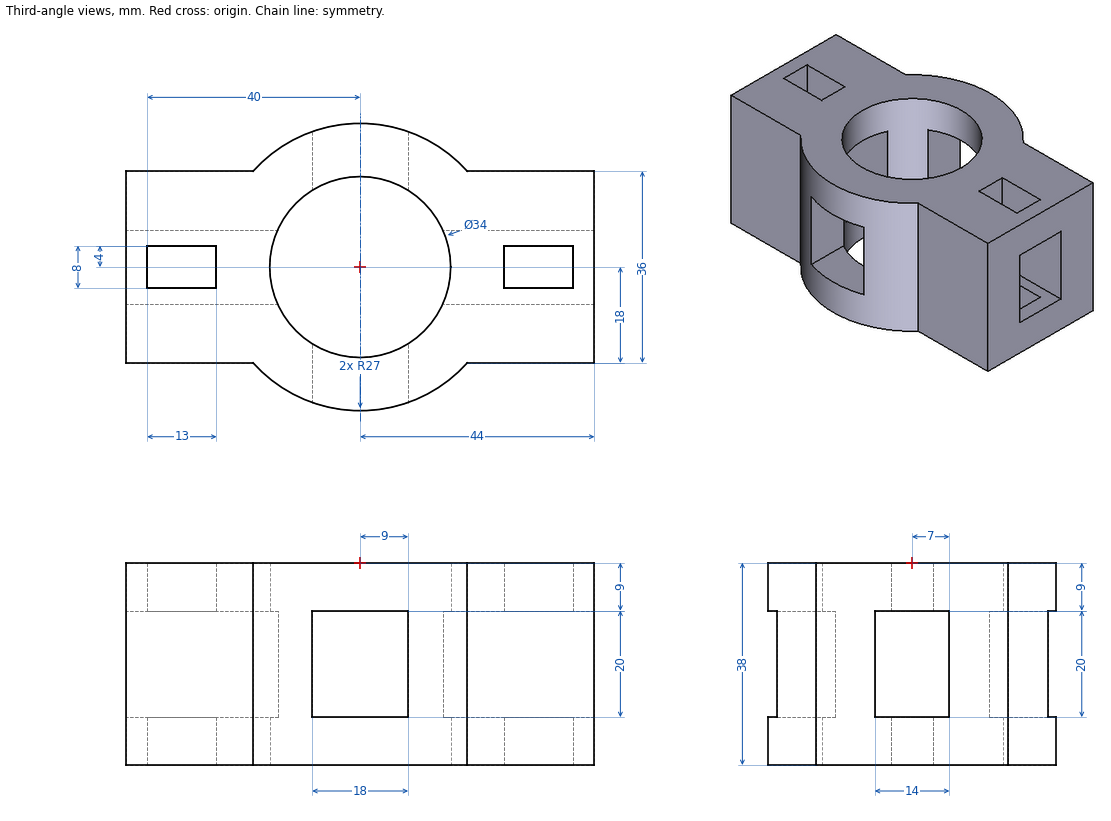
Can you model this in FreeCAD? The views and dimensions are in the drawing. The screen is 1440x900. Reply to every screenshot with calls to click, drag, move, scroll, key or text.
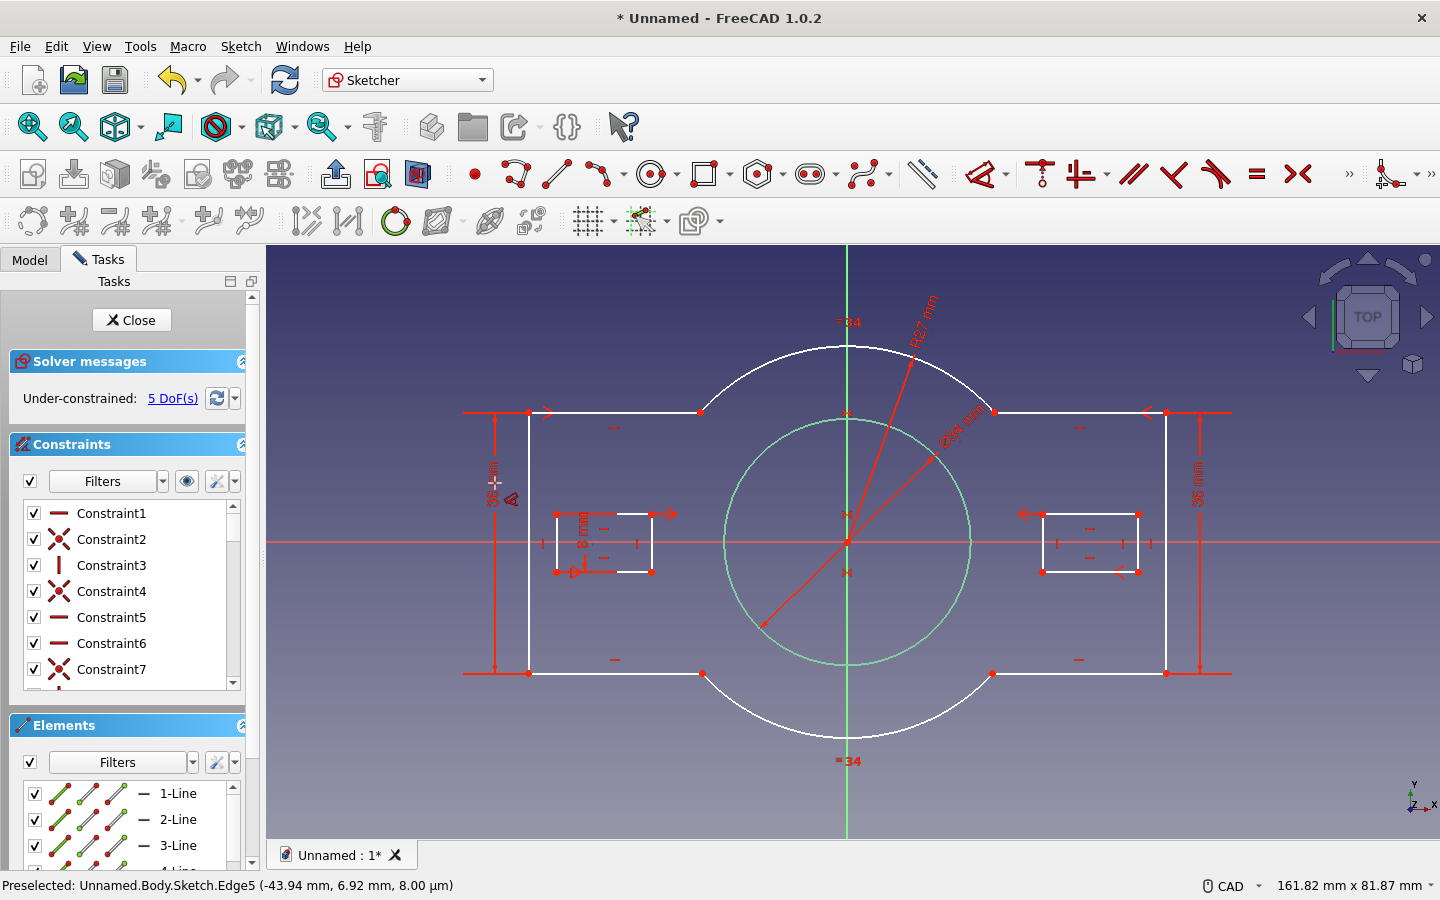
click(585, 572)
click(604, 606)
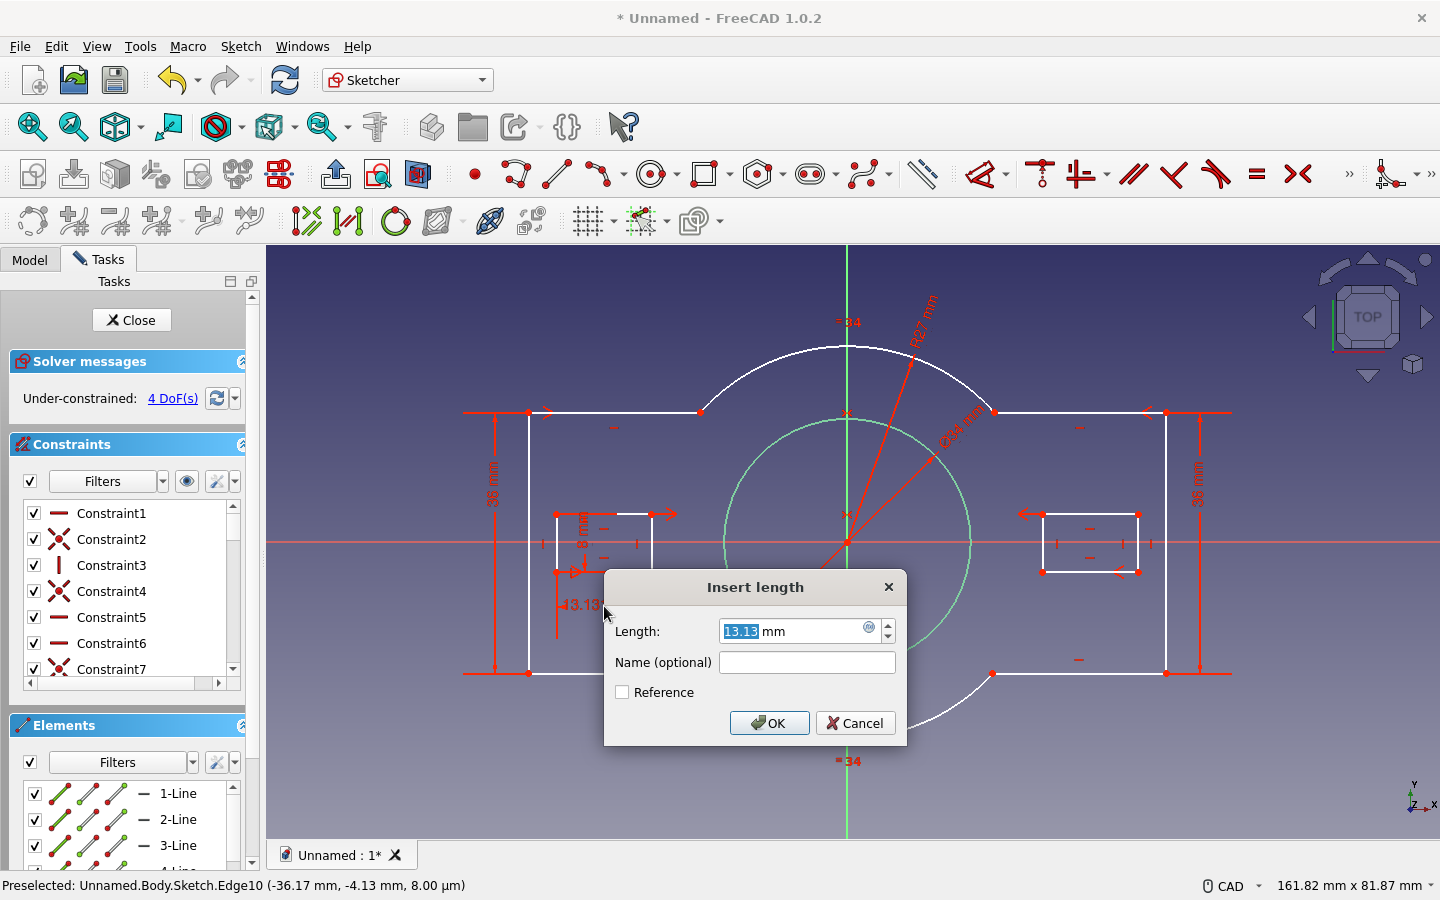
text(13)
key(Return)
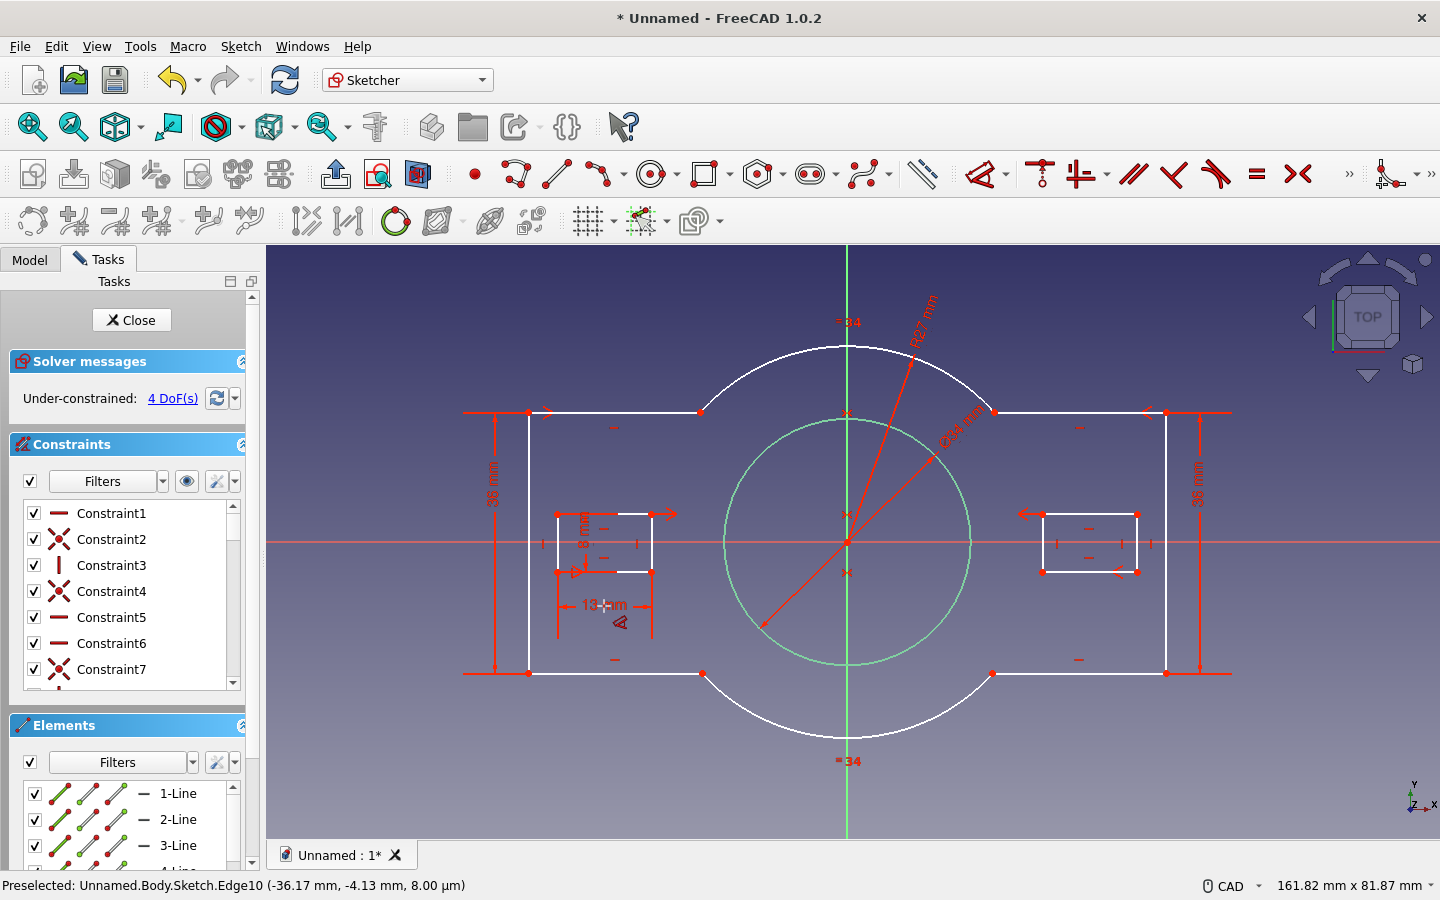
scroll(558, 514, up, 2)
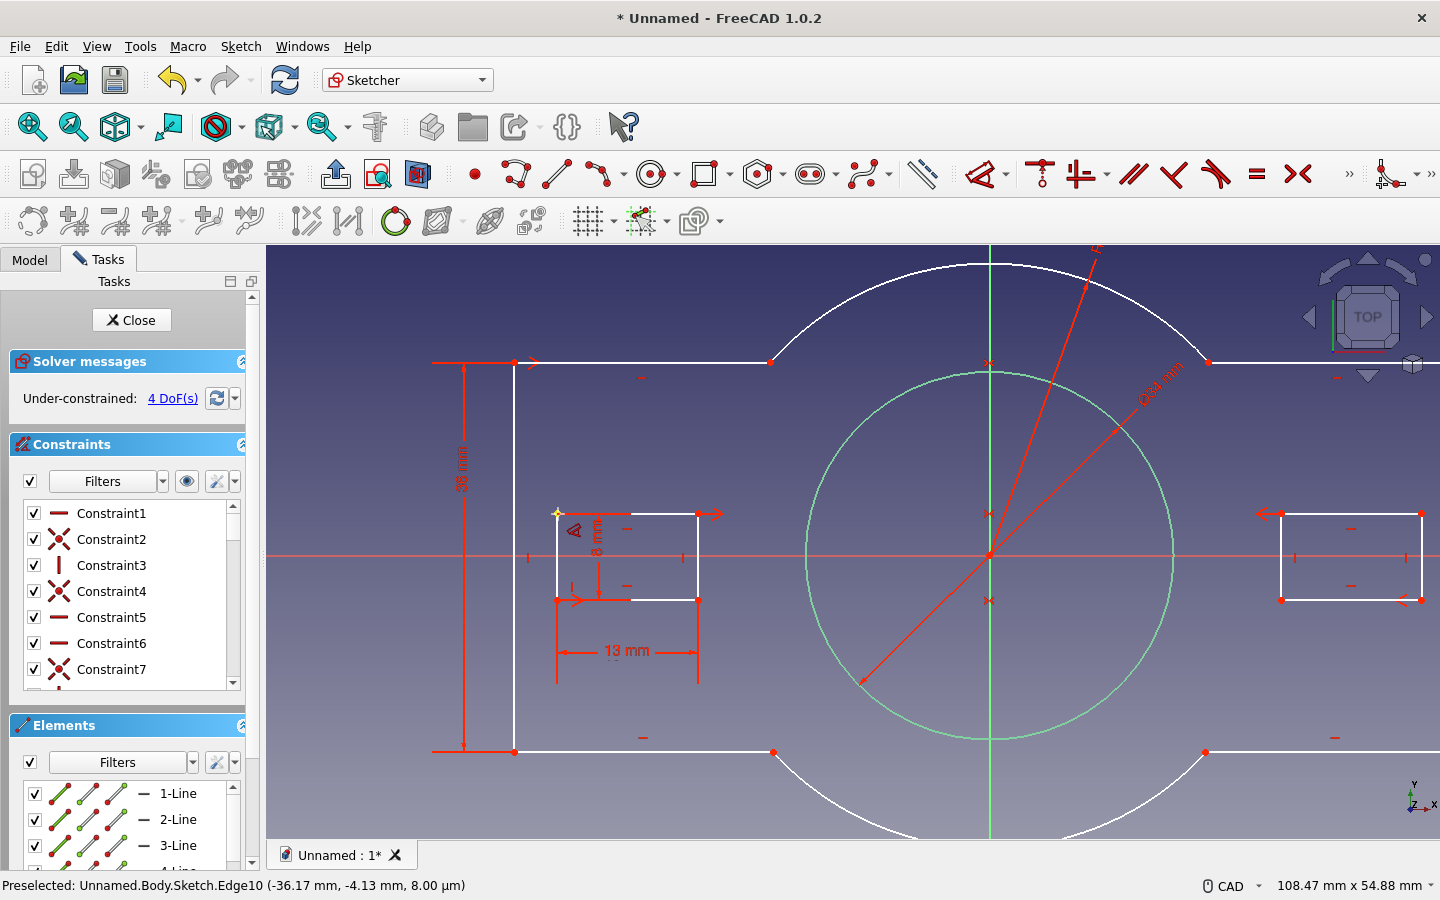
click(557, 514)
click(1024, 535)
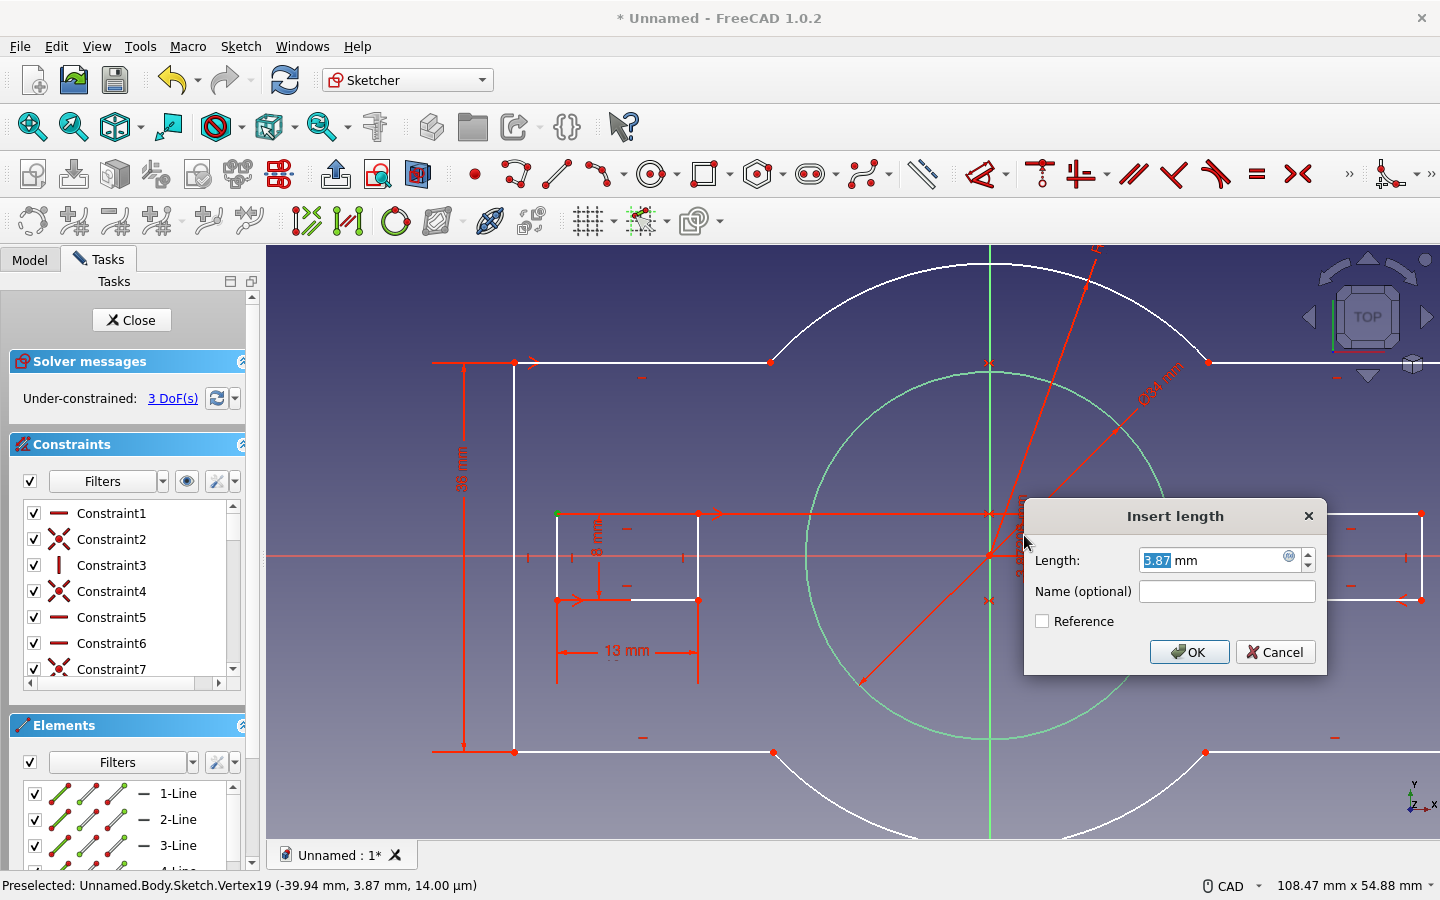
text(4)
key(Return)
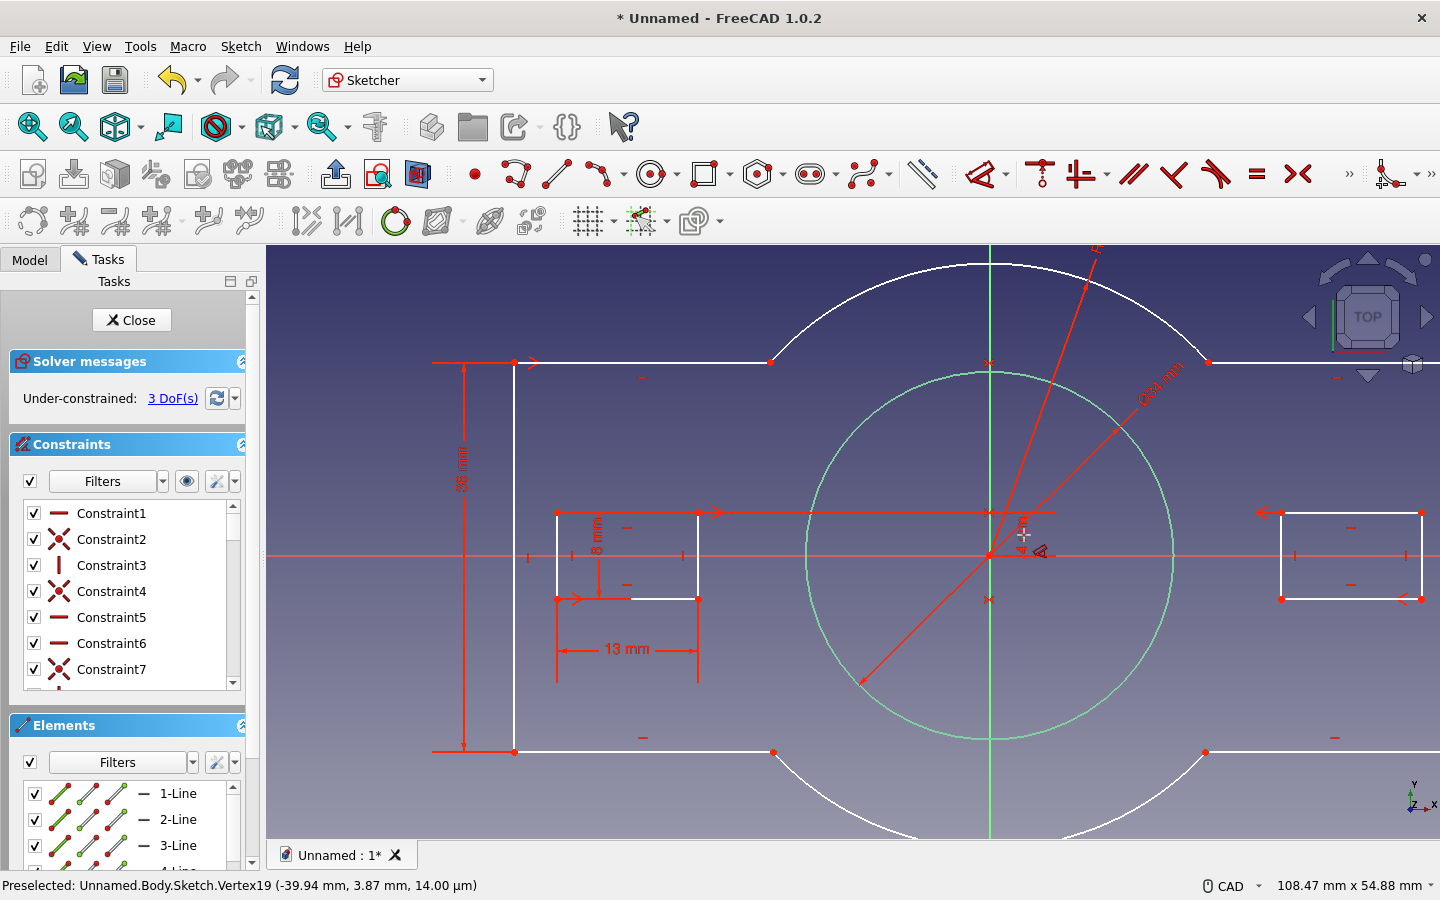
click(1206, 752)
click(1240, 654)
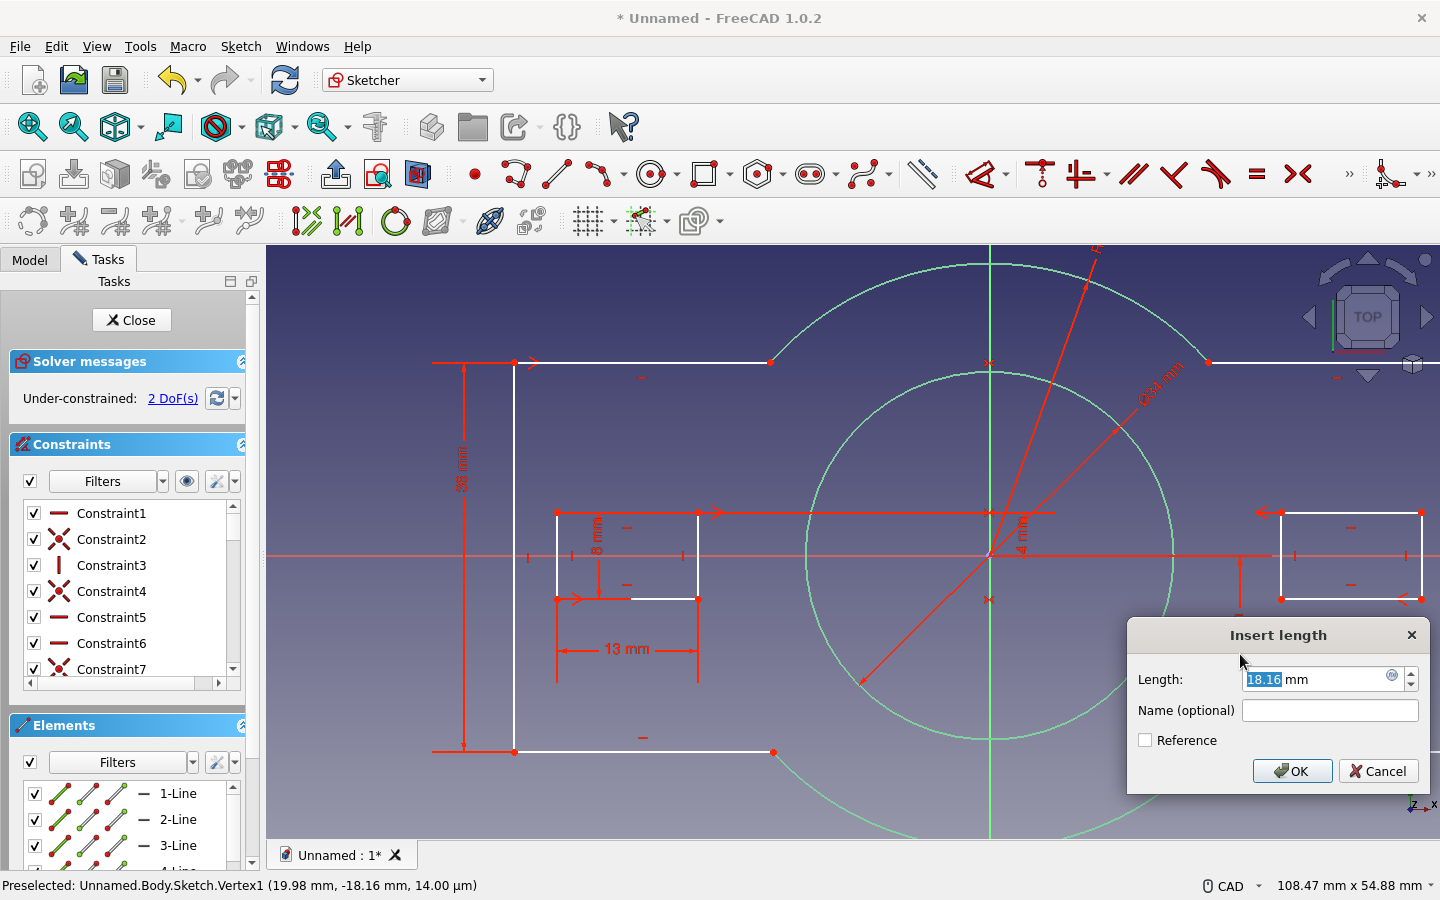
text(18)
key(Return)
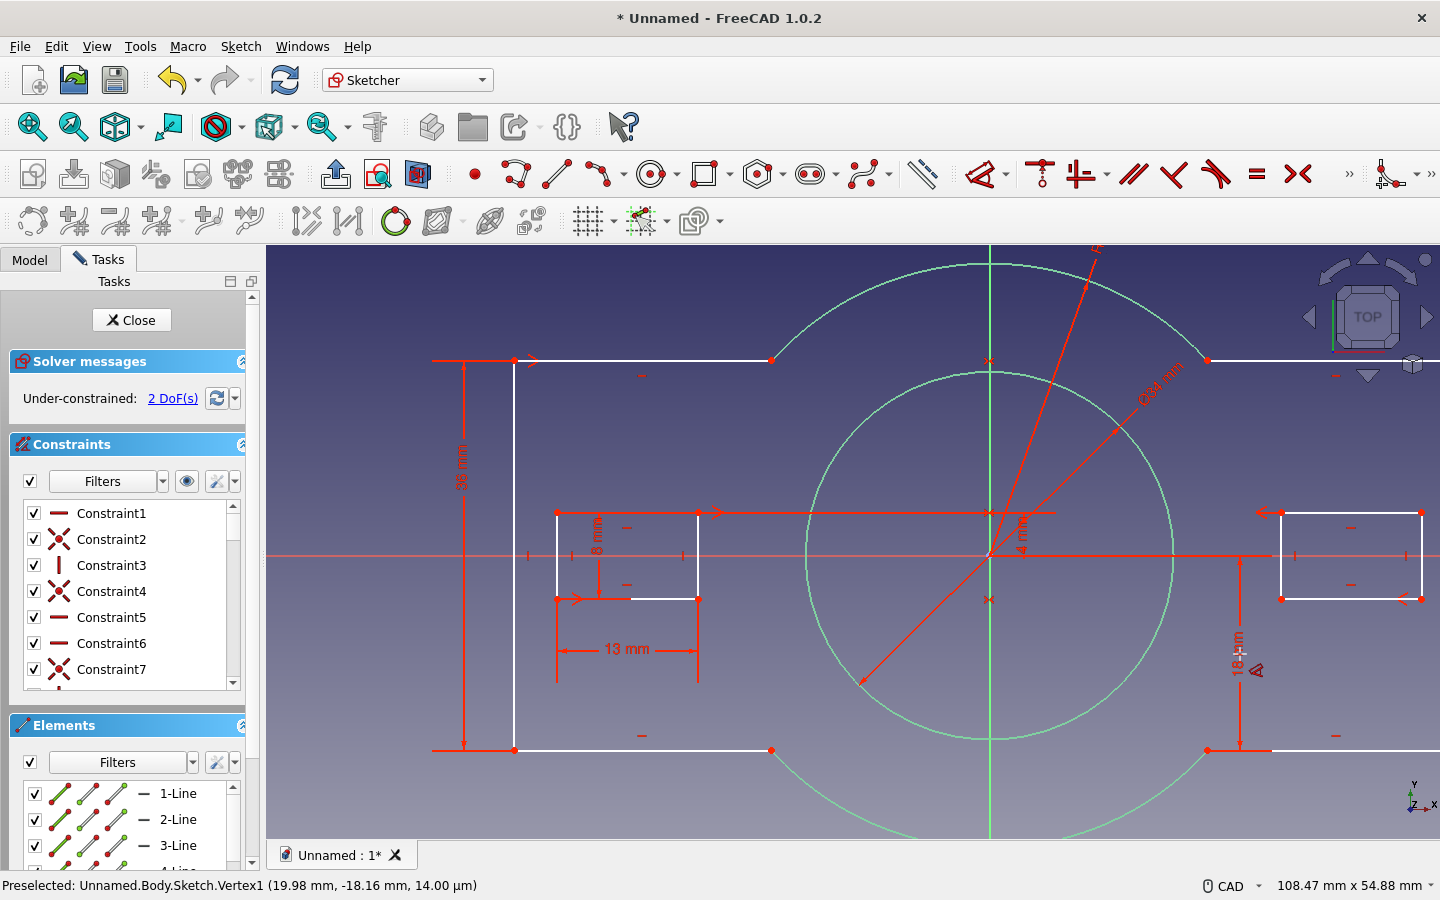
scroll(367, 514, down, 2)